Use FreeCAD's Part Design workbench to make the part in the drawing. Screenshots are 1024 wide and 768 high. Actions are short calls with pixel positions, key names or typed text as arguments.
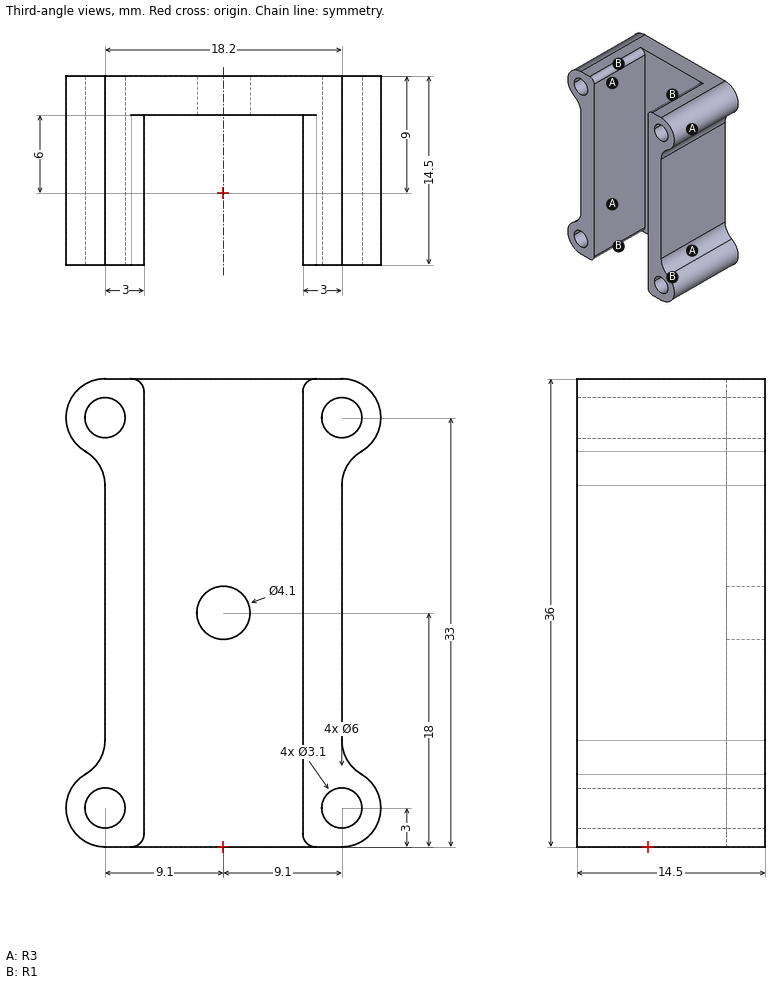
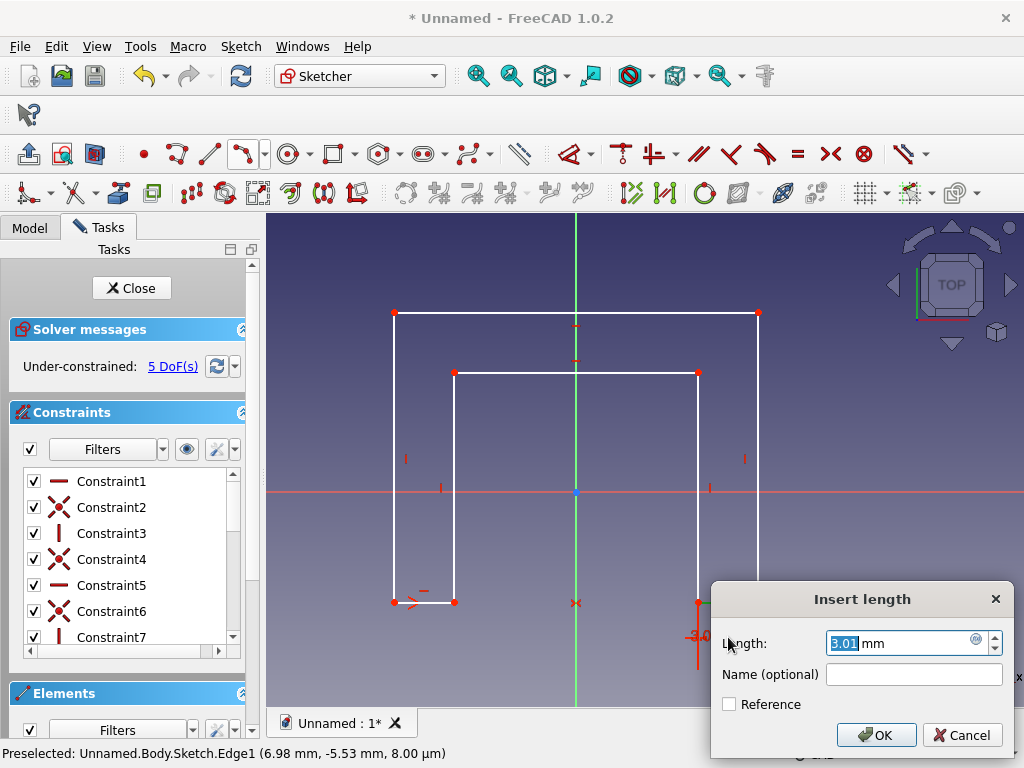
text(3)
key(Return)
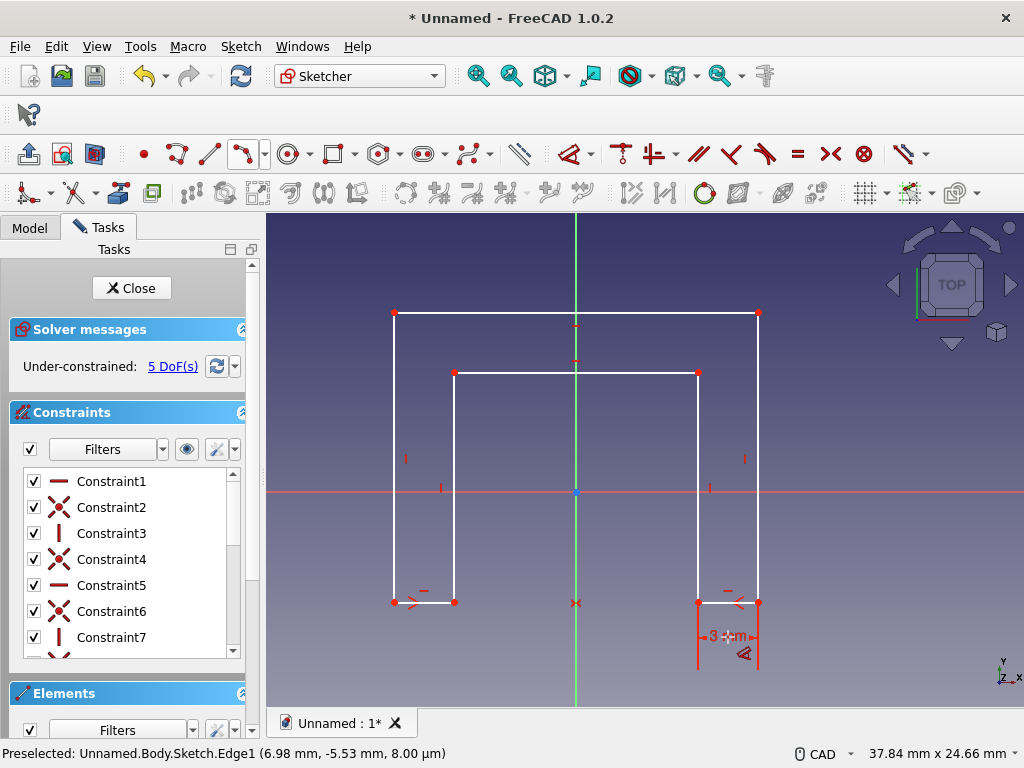
click(412, 603)
click(424, 637)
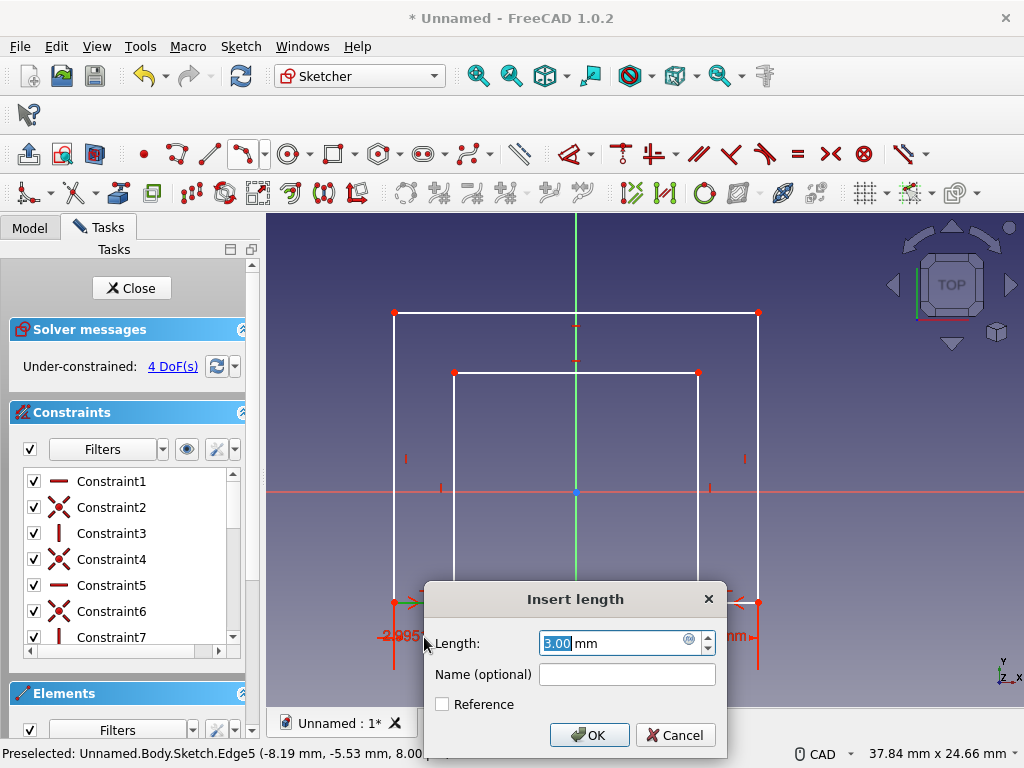
text(3)
key(Return)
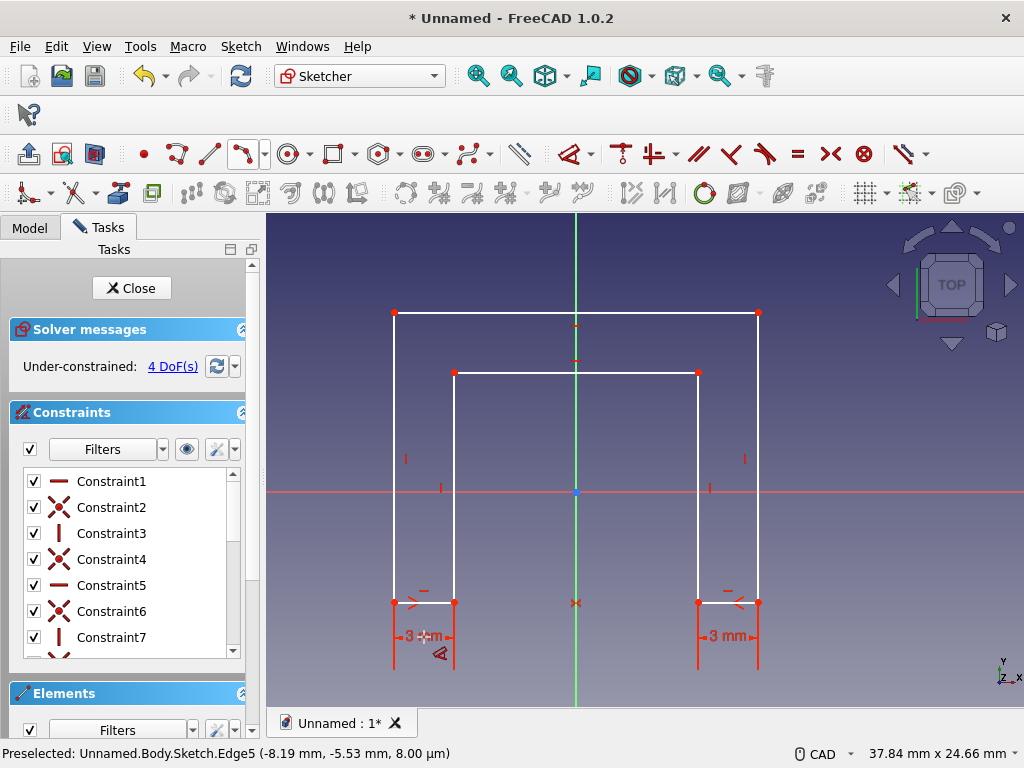
click(758, 313)
click(792, 403)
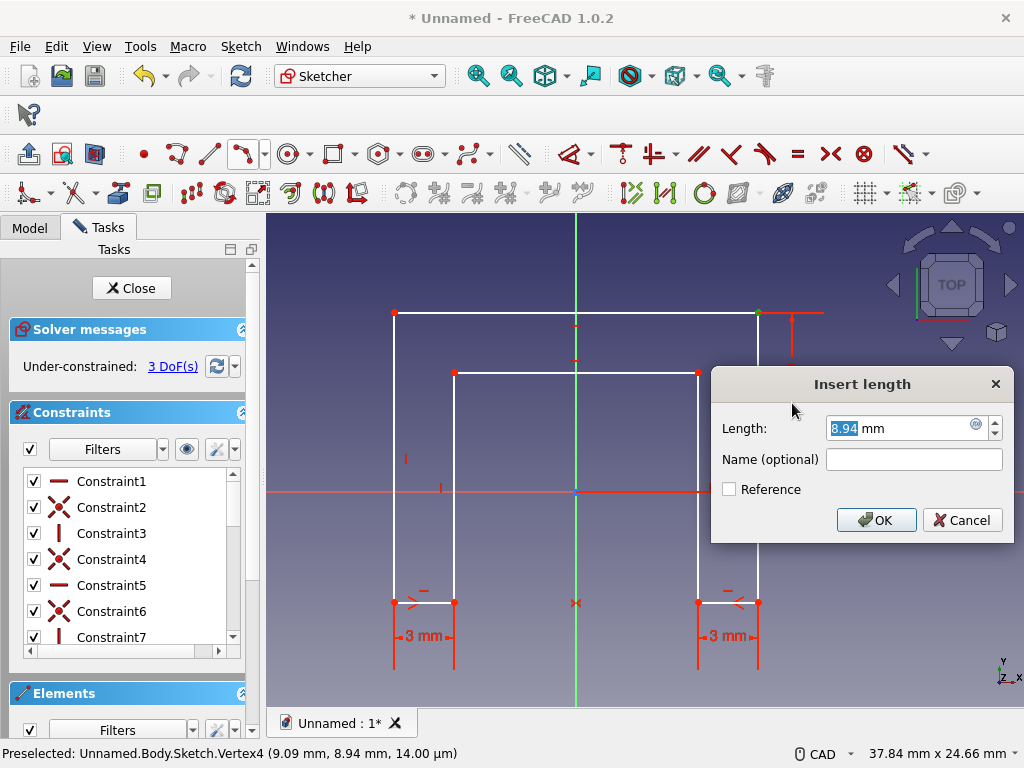
text(9)
key(Return)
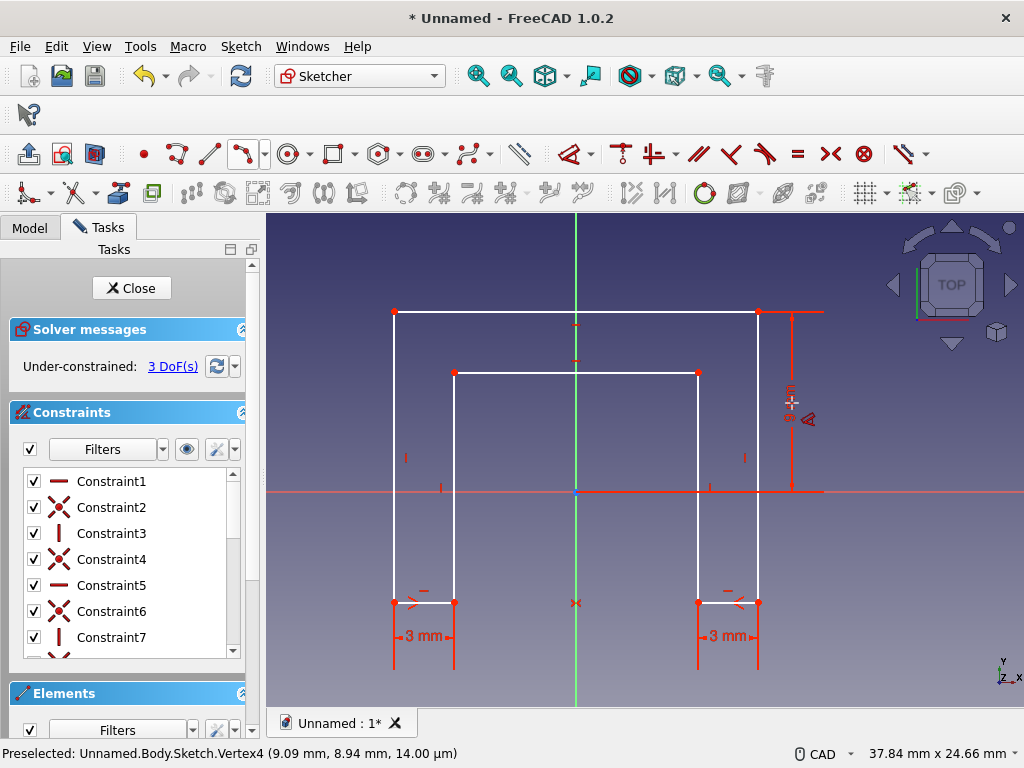
click(454, 373)
click(420, 433)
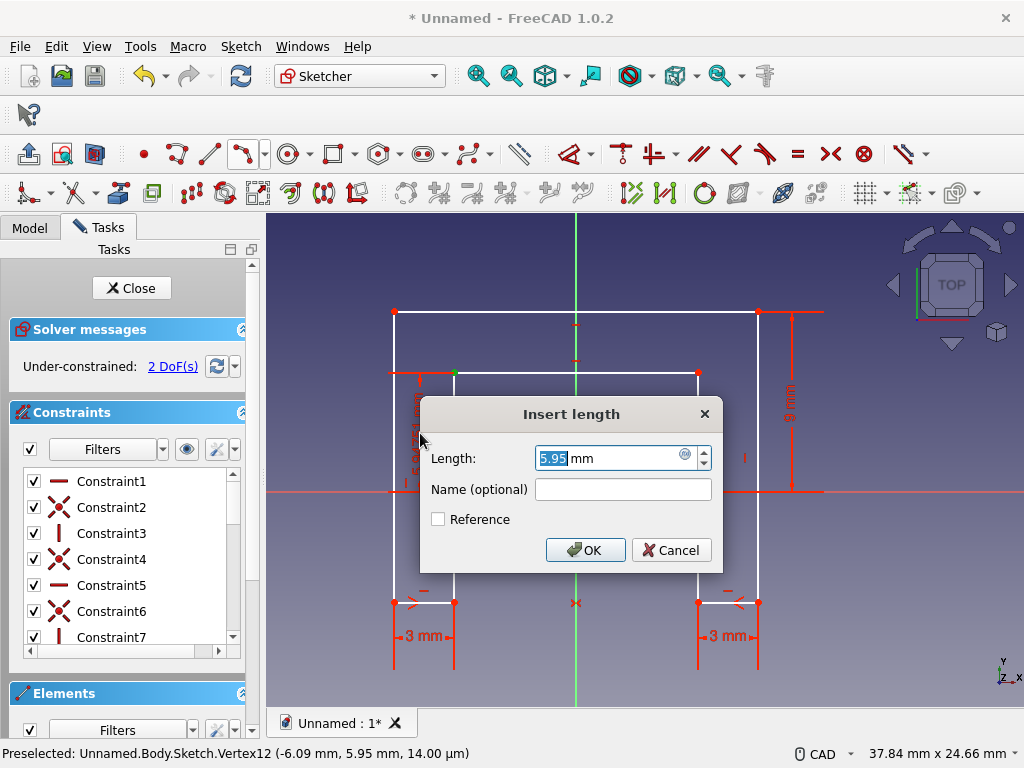
text(6)
key(Return)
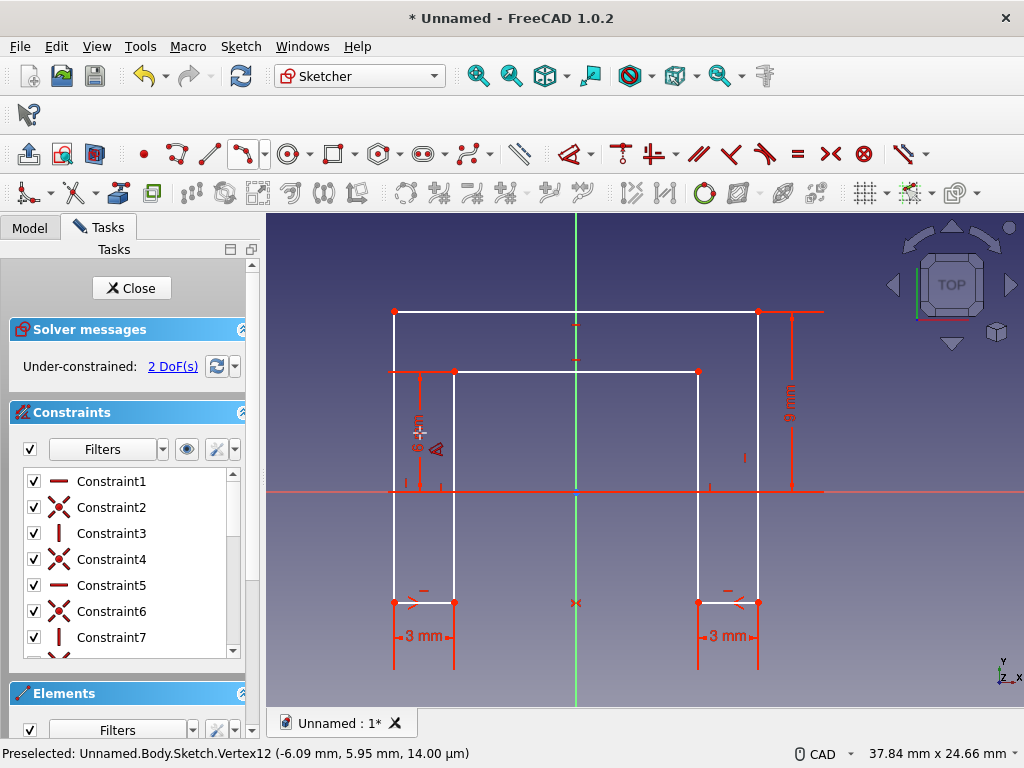
click(758, 516)
click(792, 457)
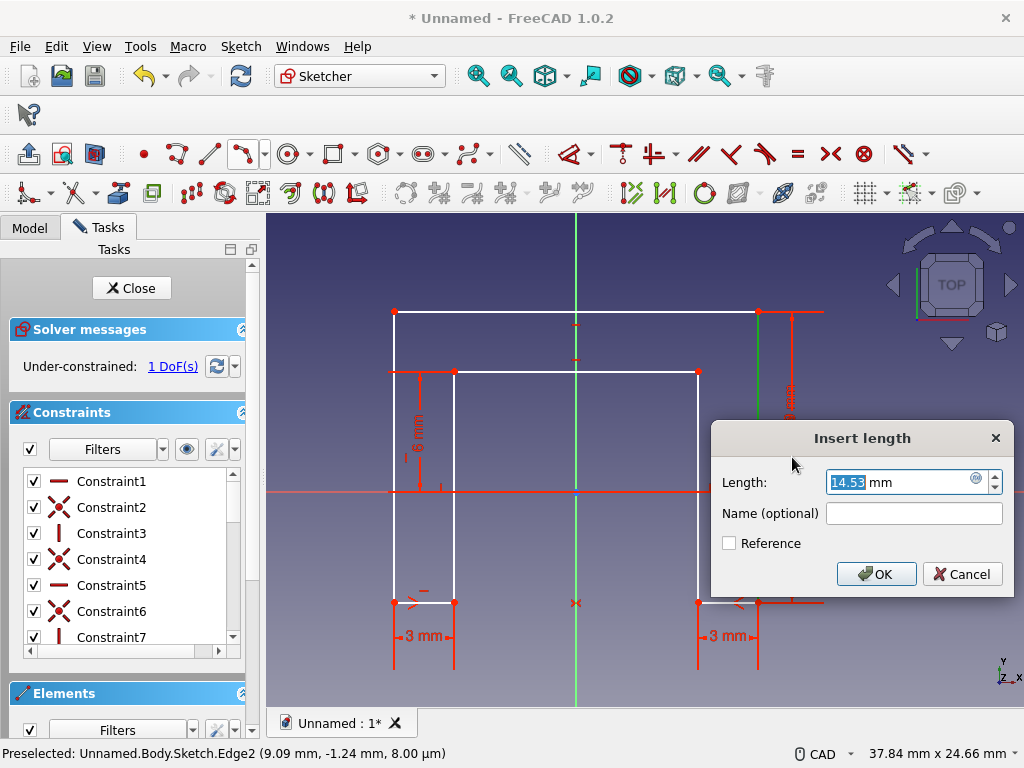
text(14.5)
key(Return)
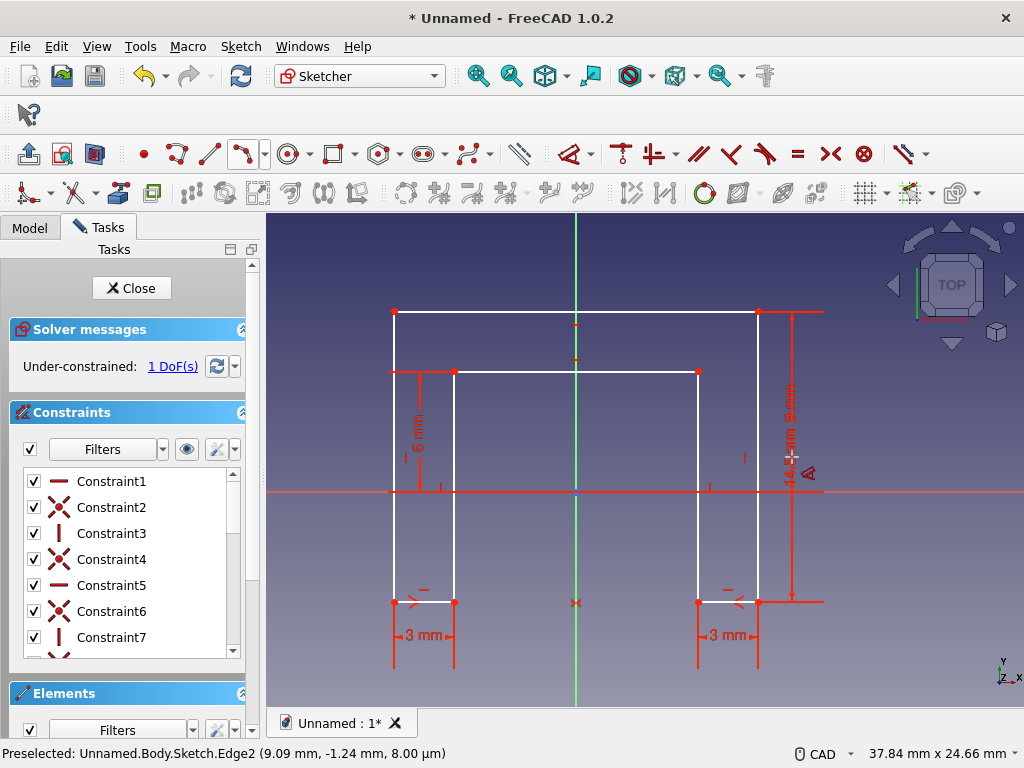
click(649, 312)
click(492, 278)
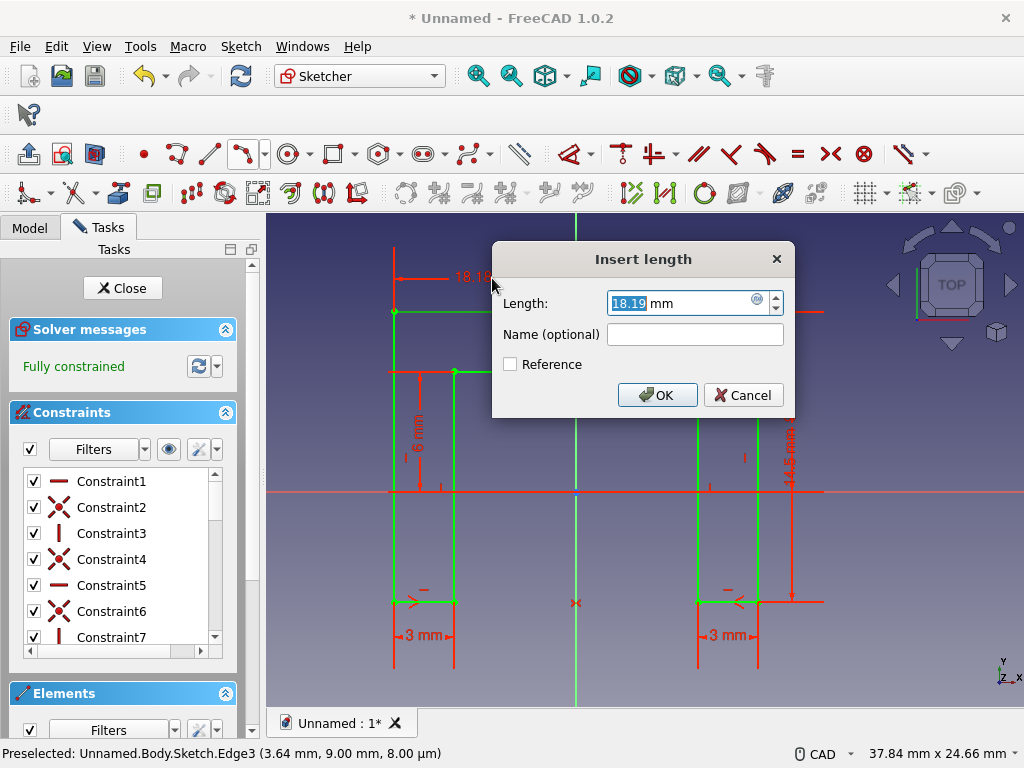
text(18.2)
key(Return)
key(Escape)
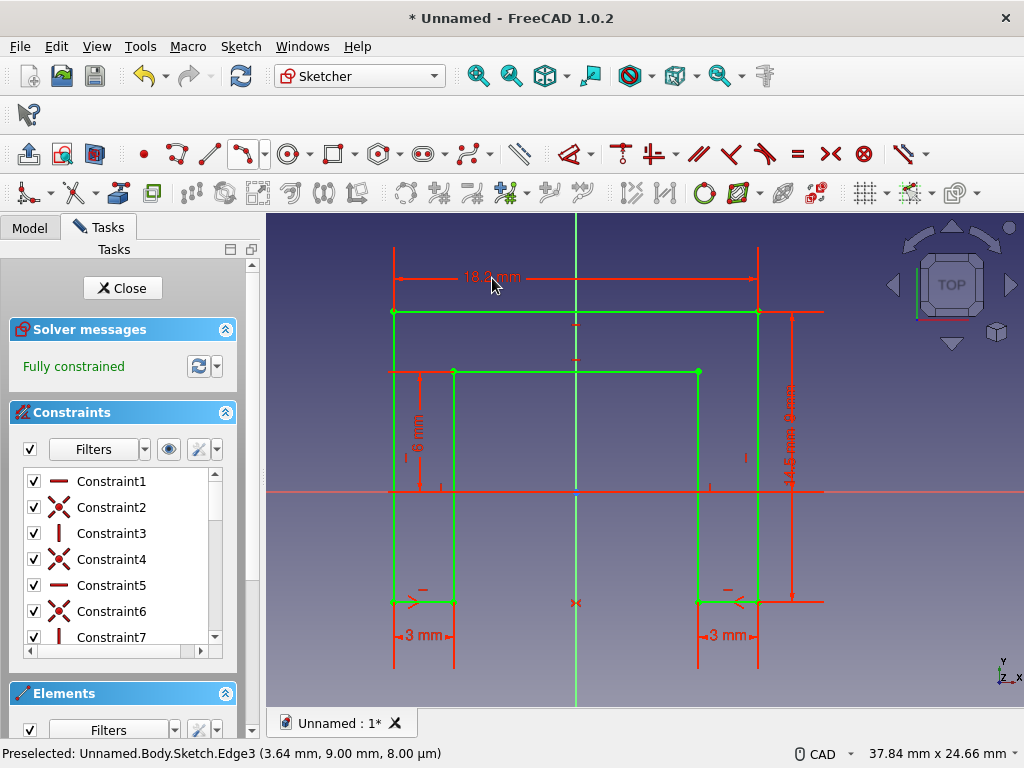
click(123, 288)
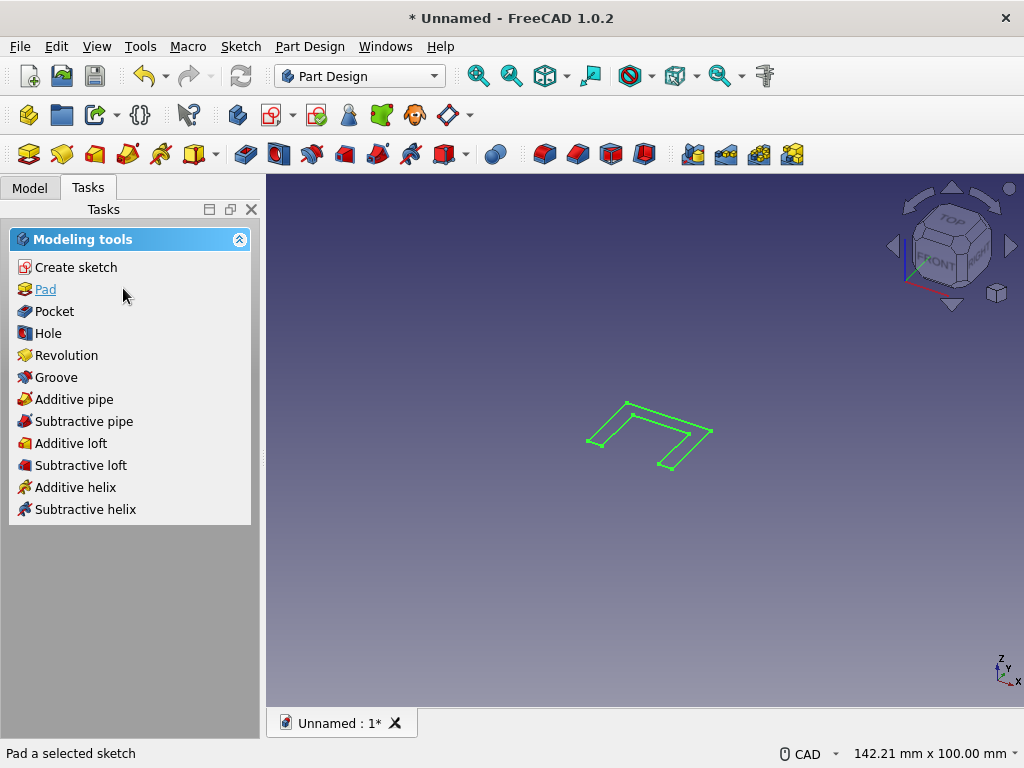
click(29, 154)